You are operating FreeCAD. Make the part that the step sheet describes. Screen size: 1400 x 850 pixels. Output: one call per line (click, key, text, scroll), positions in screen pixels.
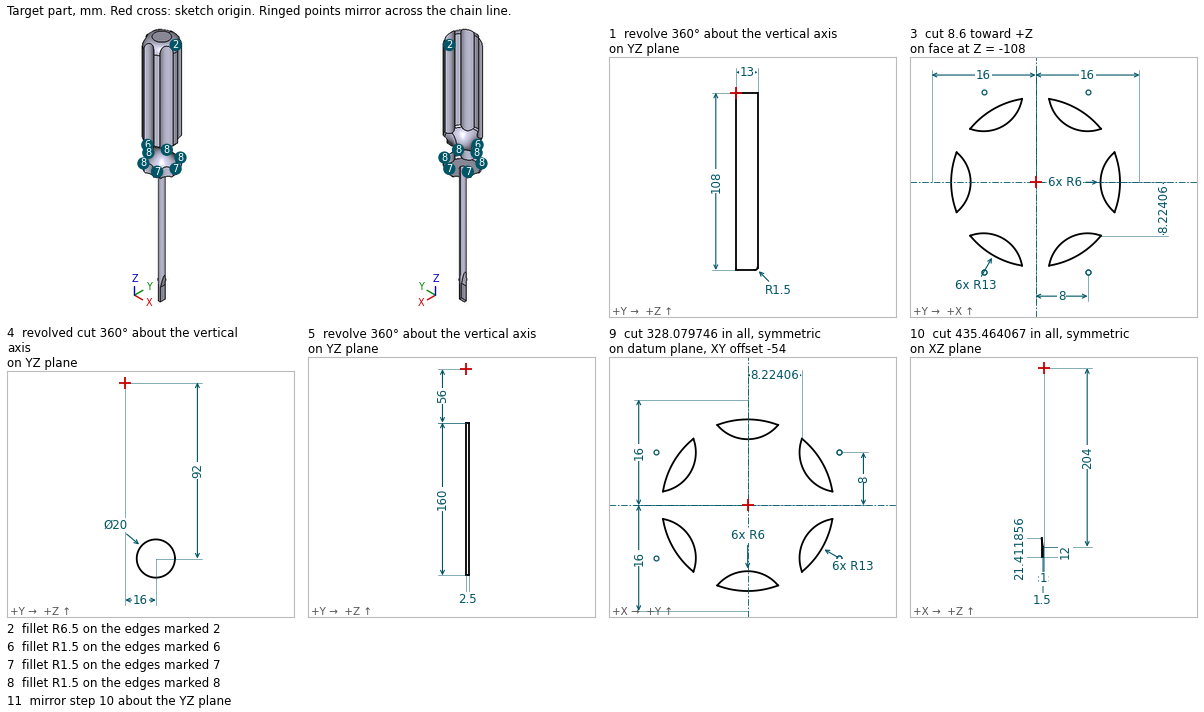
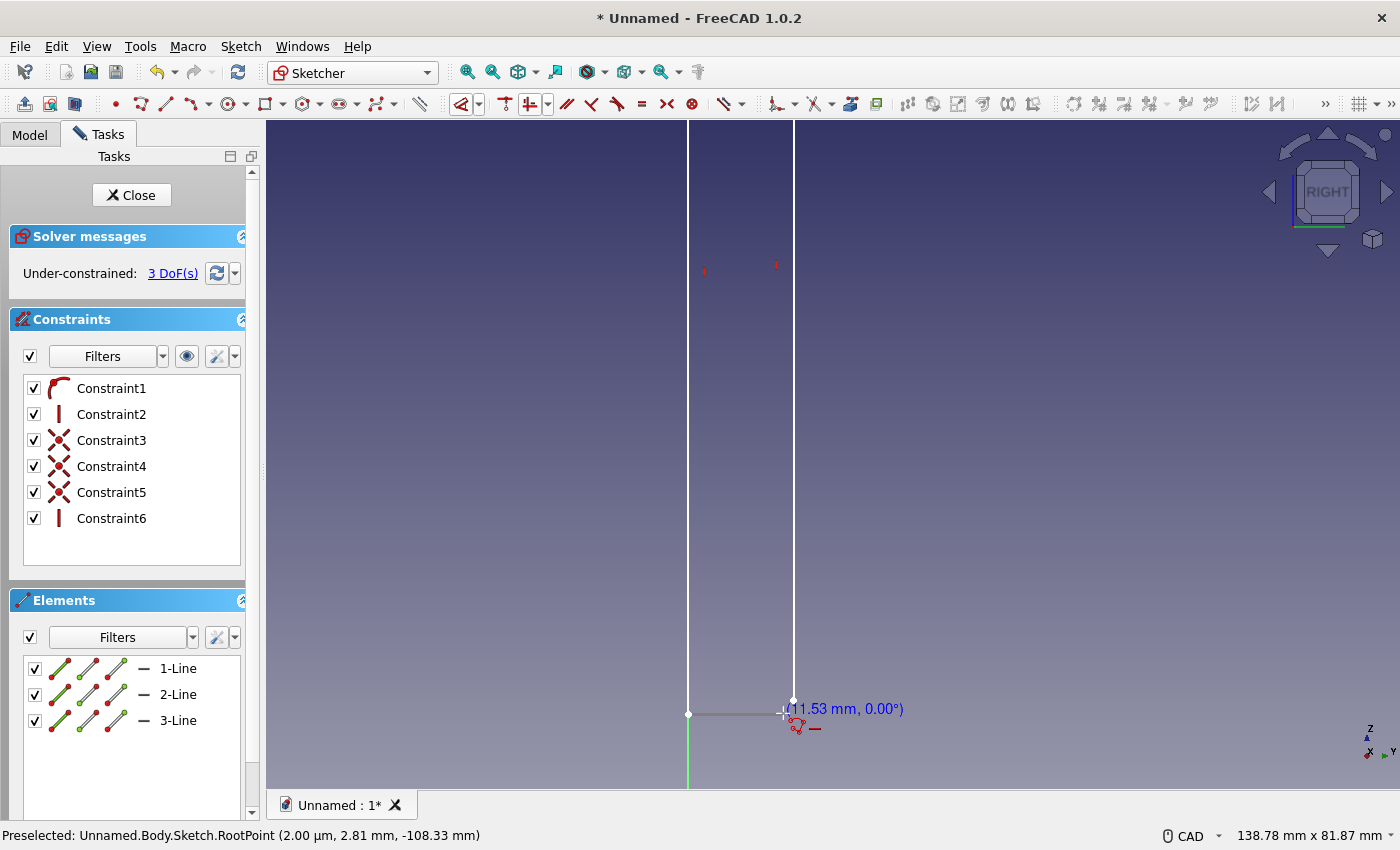
click(782, 712)
right_click(782, 712)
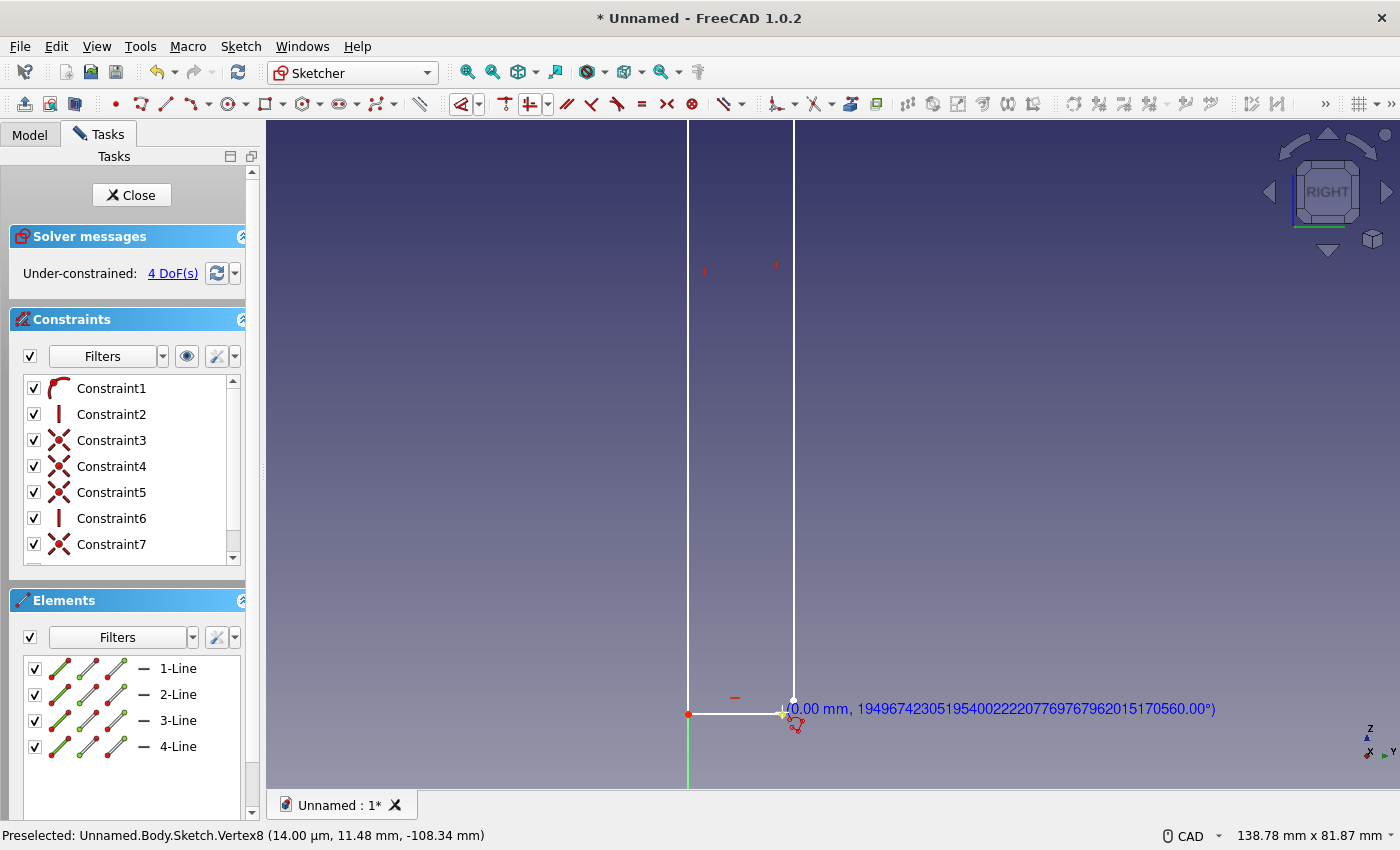
key(g)
key(3)
key(a)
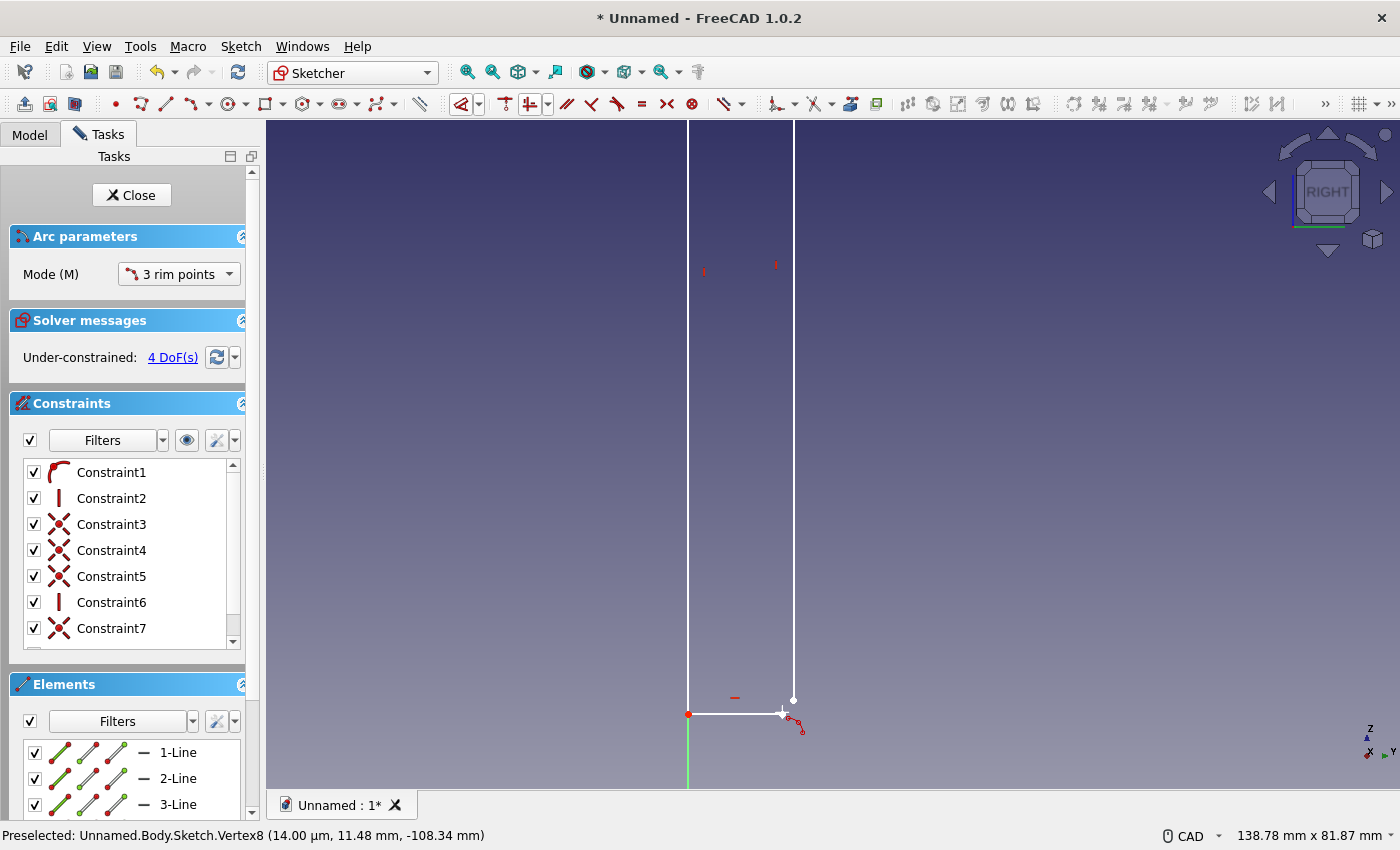
click(782, 714)
click(794, 701)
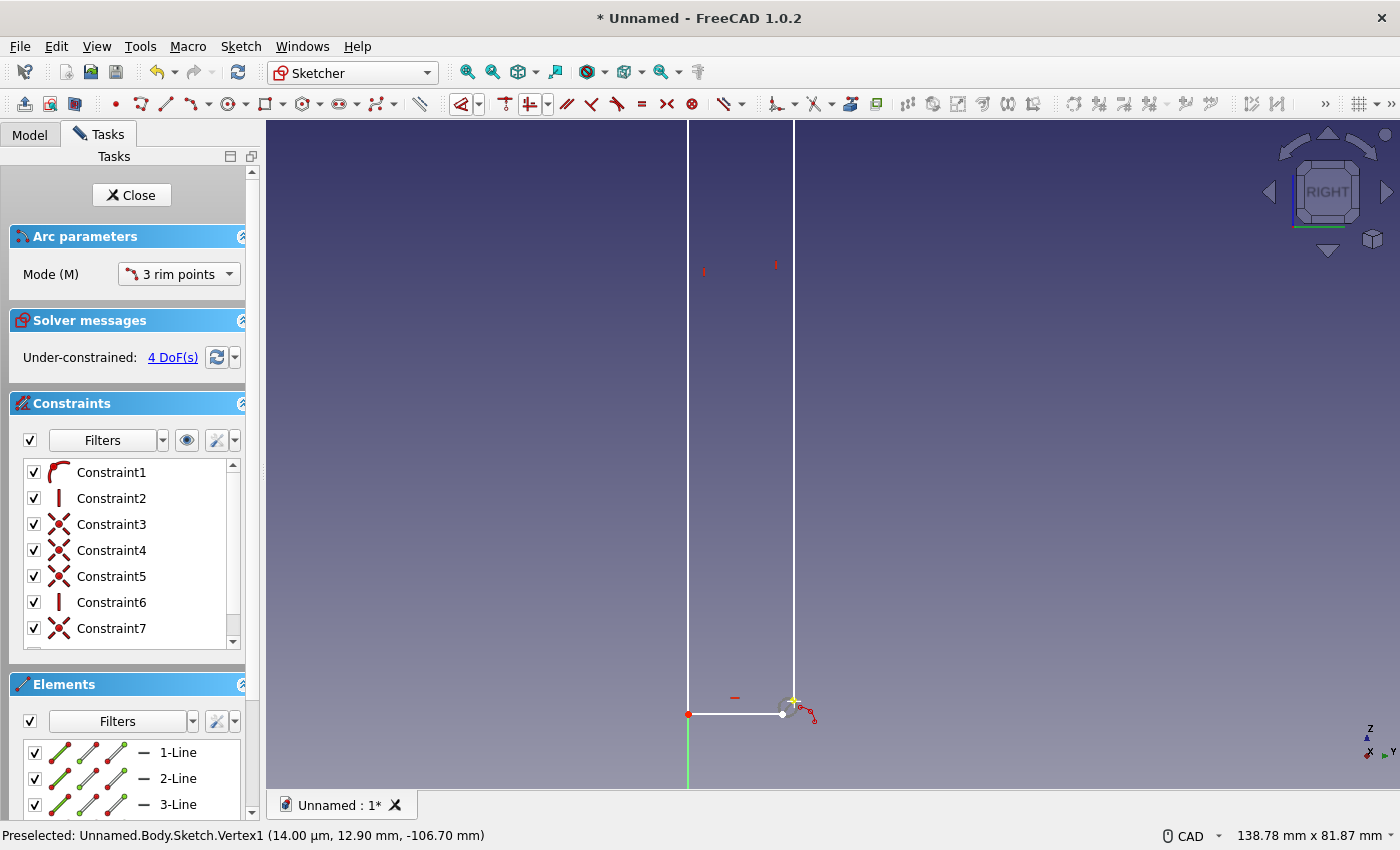
scroll(791, 708, up, 8)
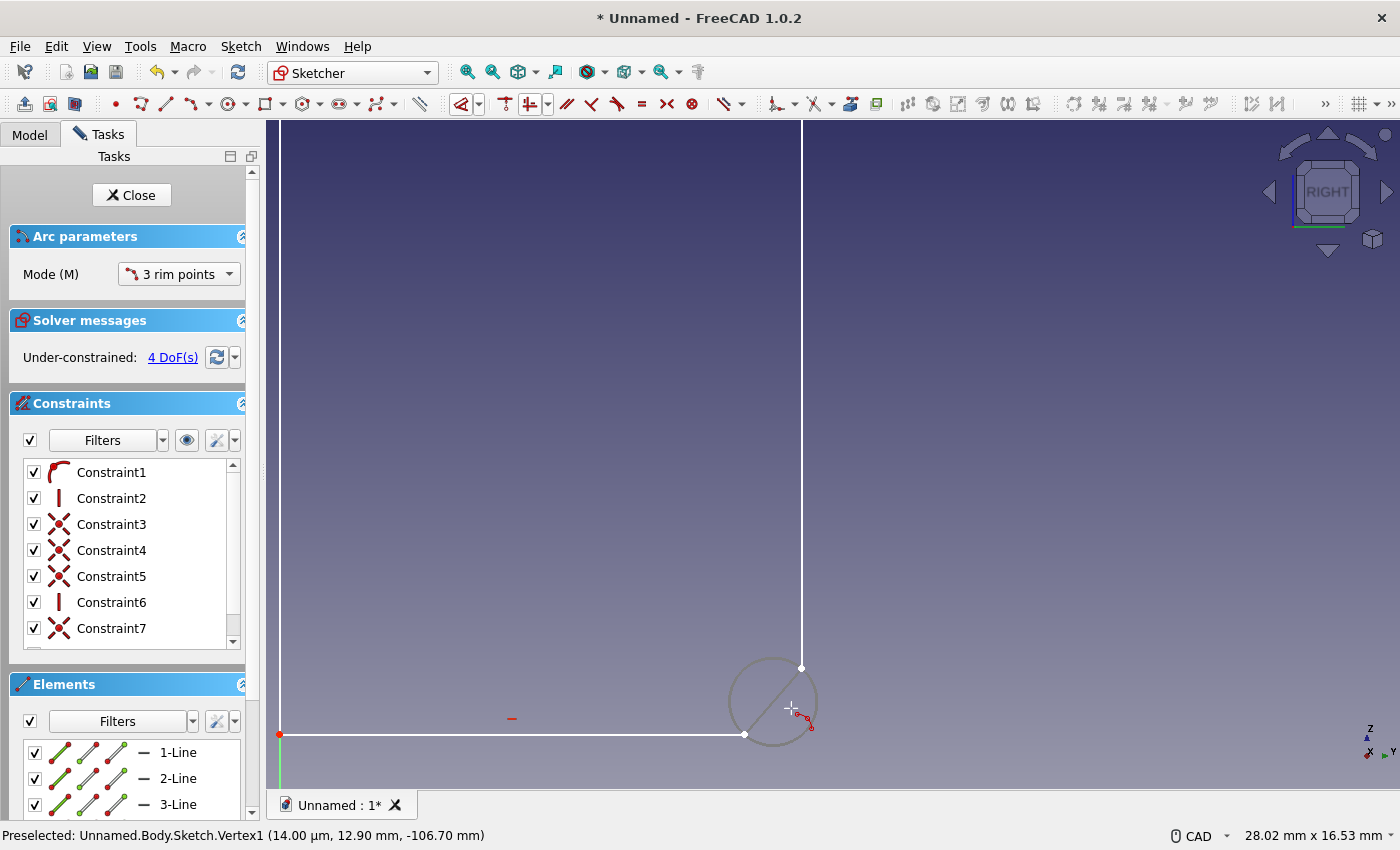
click(788, 703)
key(Escape)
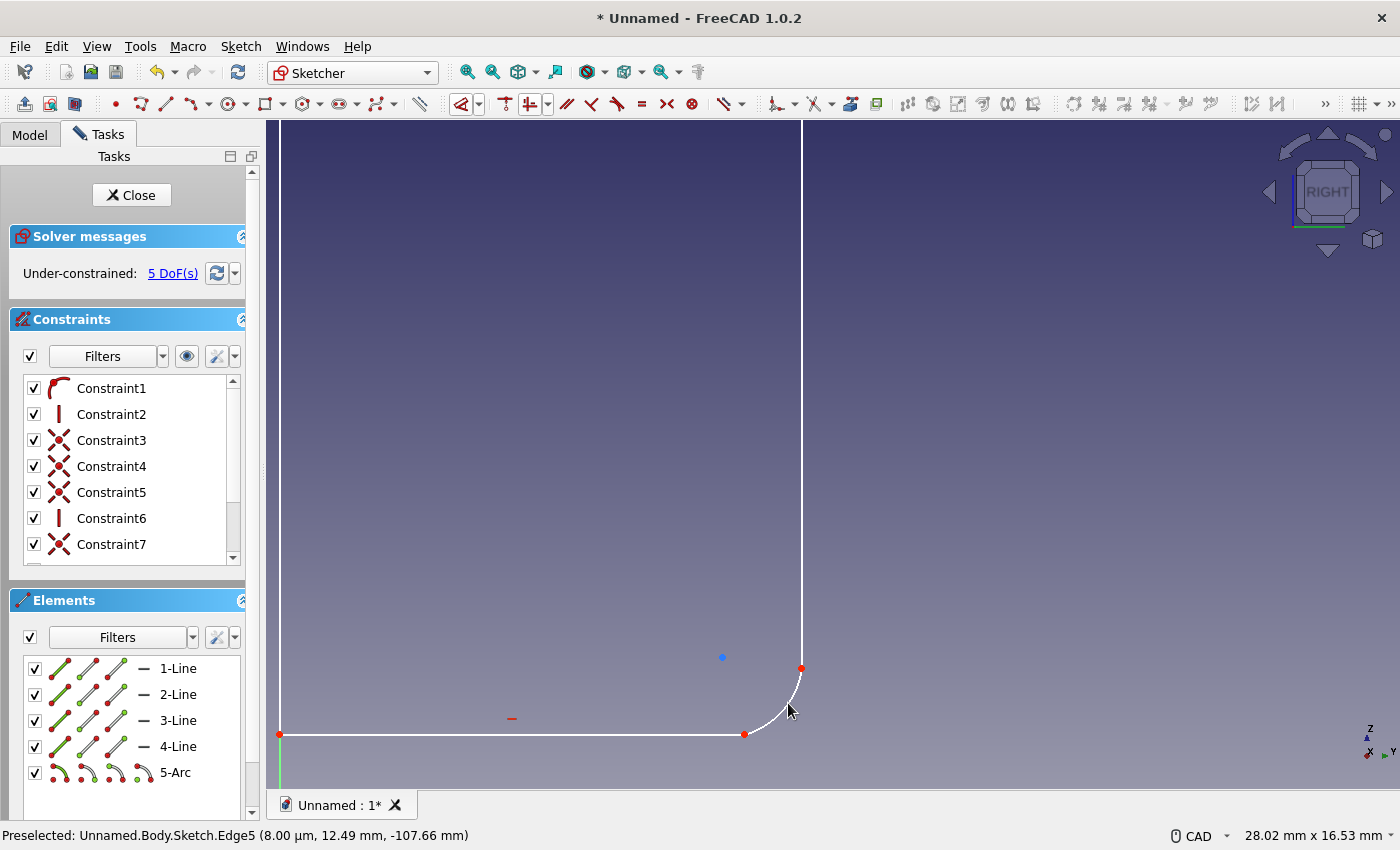
scroll(787, 646, down, 12)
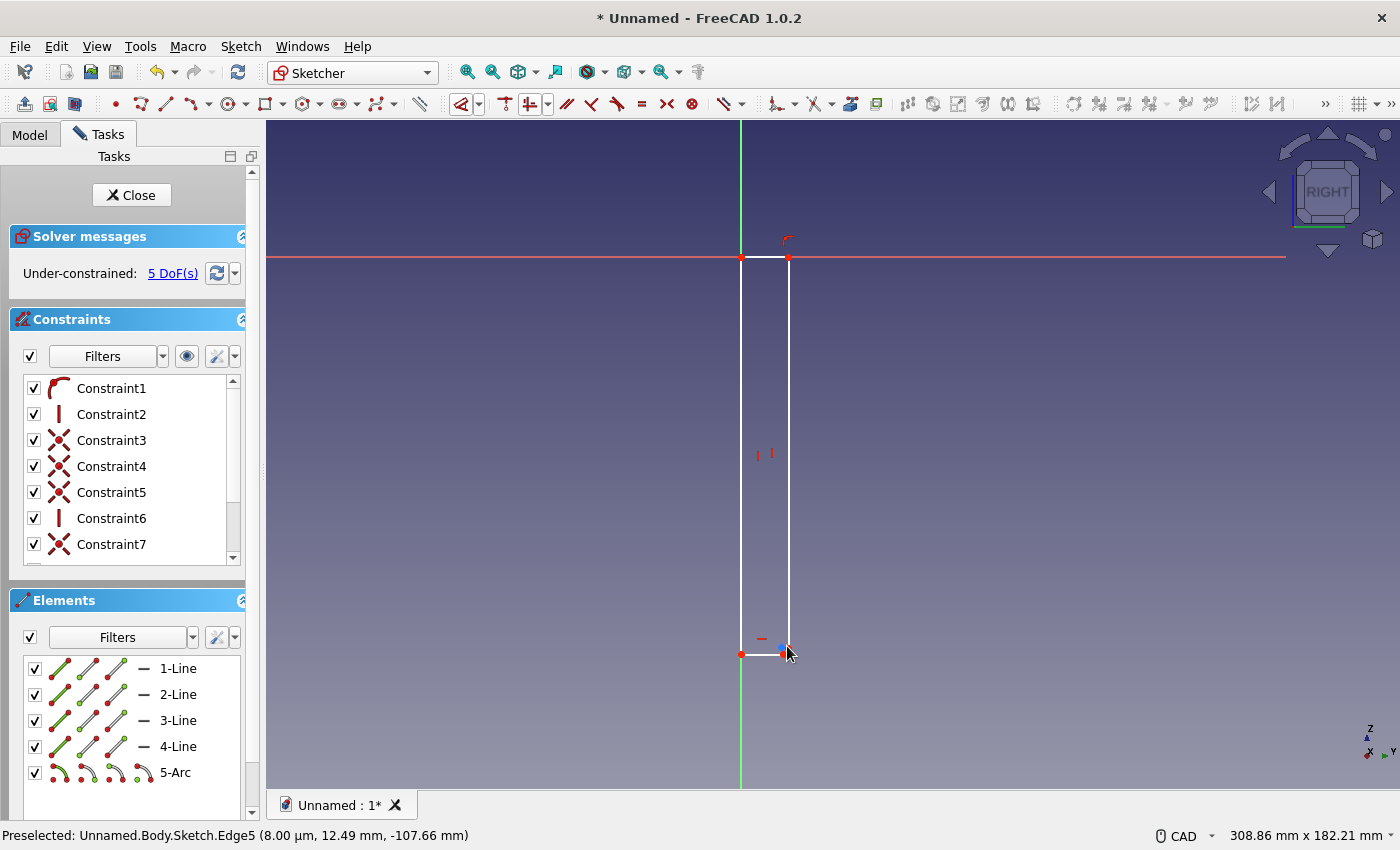
click(789, 531)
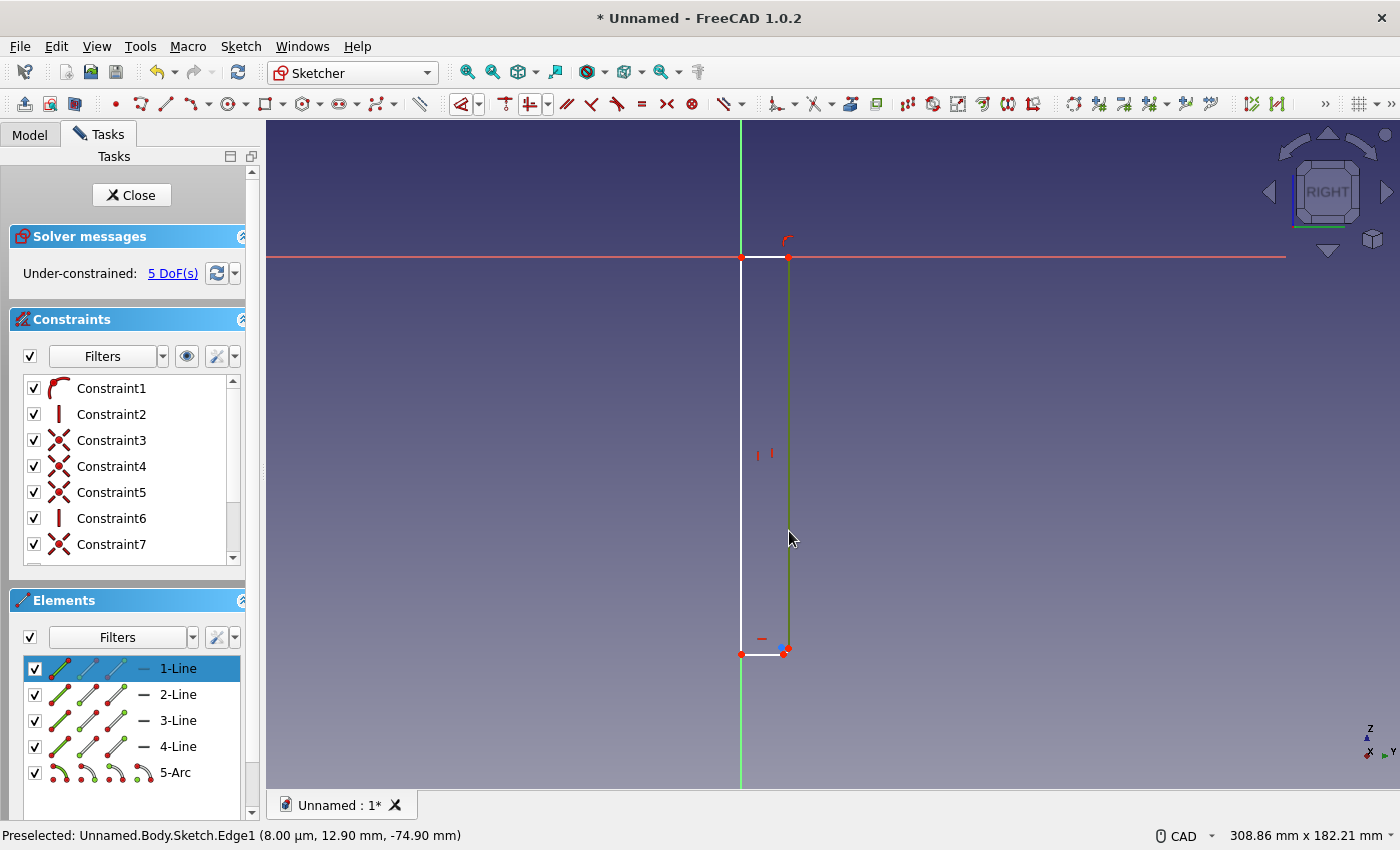
scroll(787, 653, up, 7)